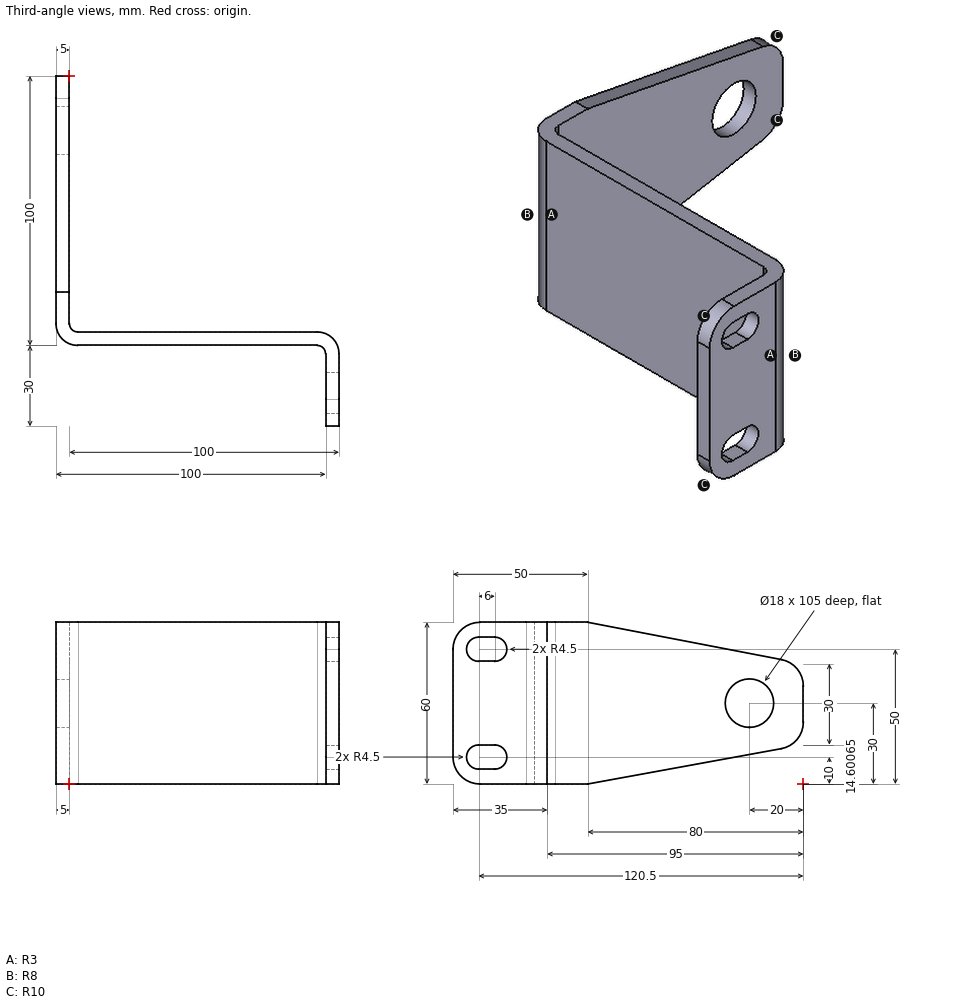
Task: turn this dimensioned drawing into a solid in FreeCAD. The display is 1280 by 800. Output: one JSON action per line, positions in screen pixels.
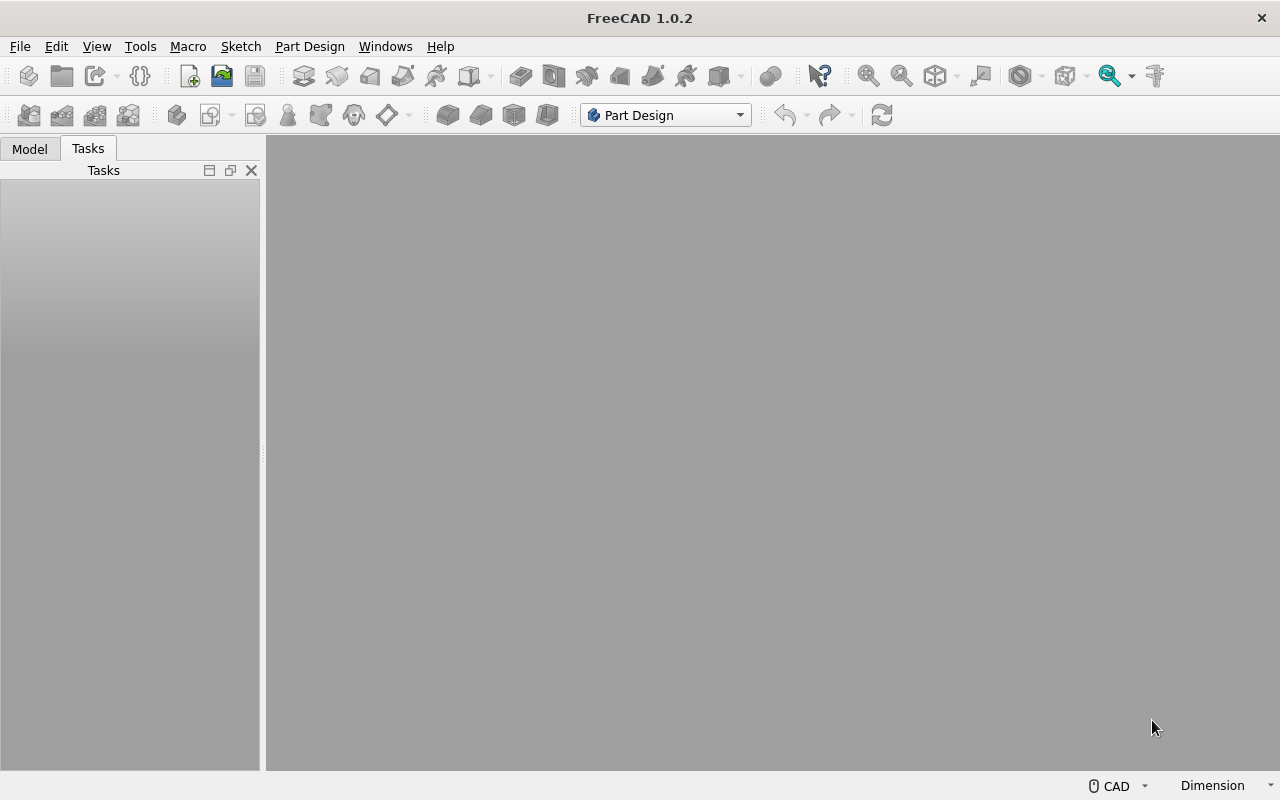
{"action": "left_click", "coordinate": [189, 76]}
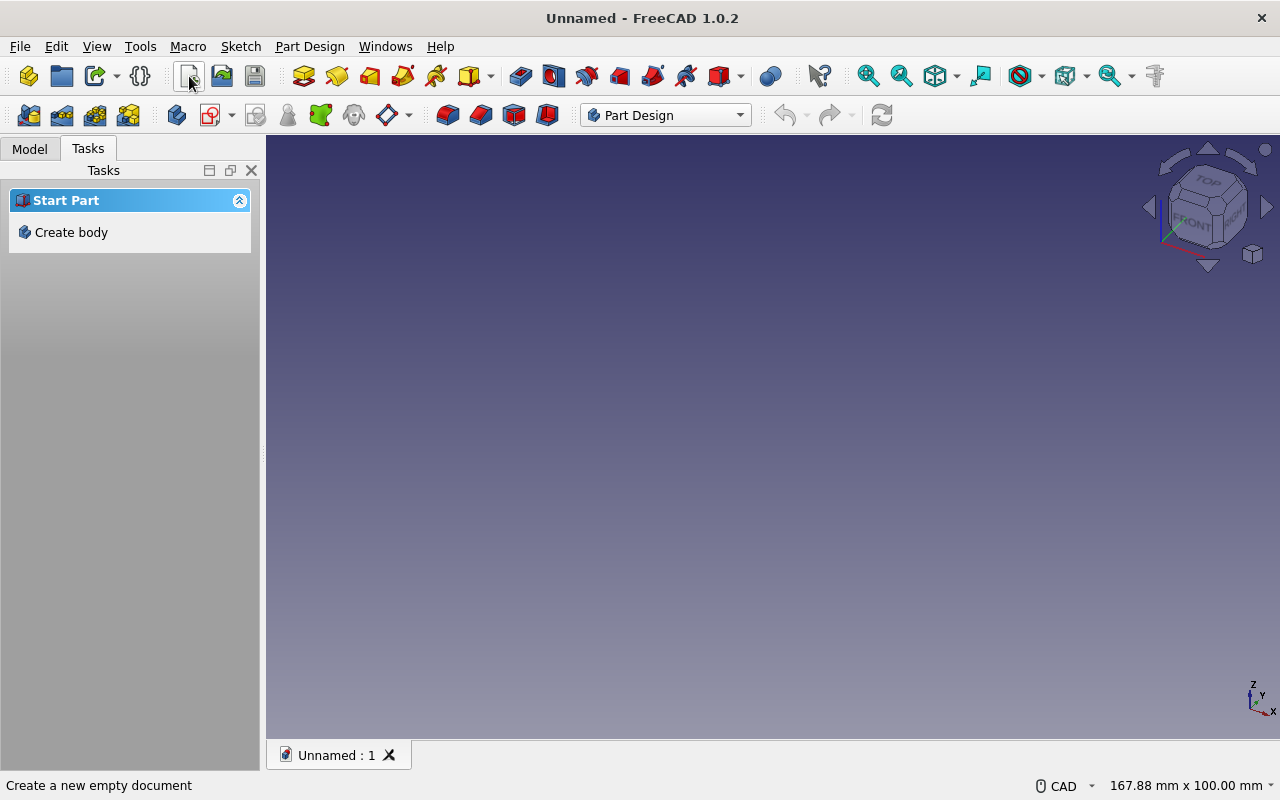
{"action": "left_click", "coordinate": [210, 116]}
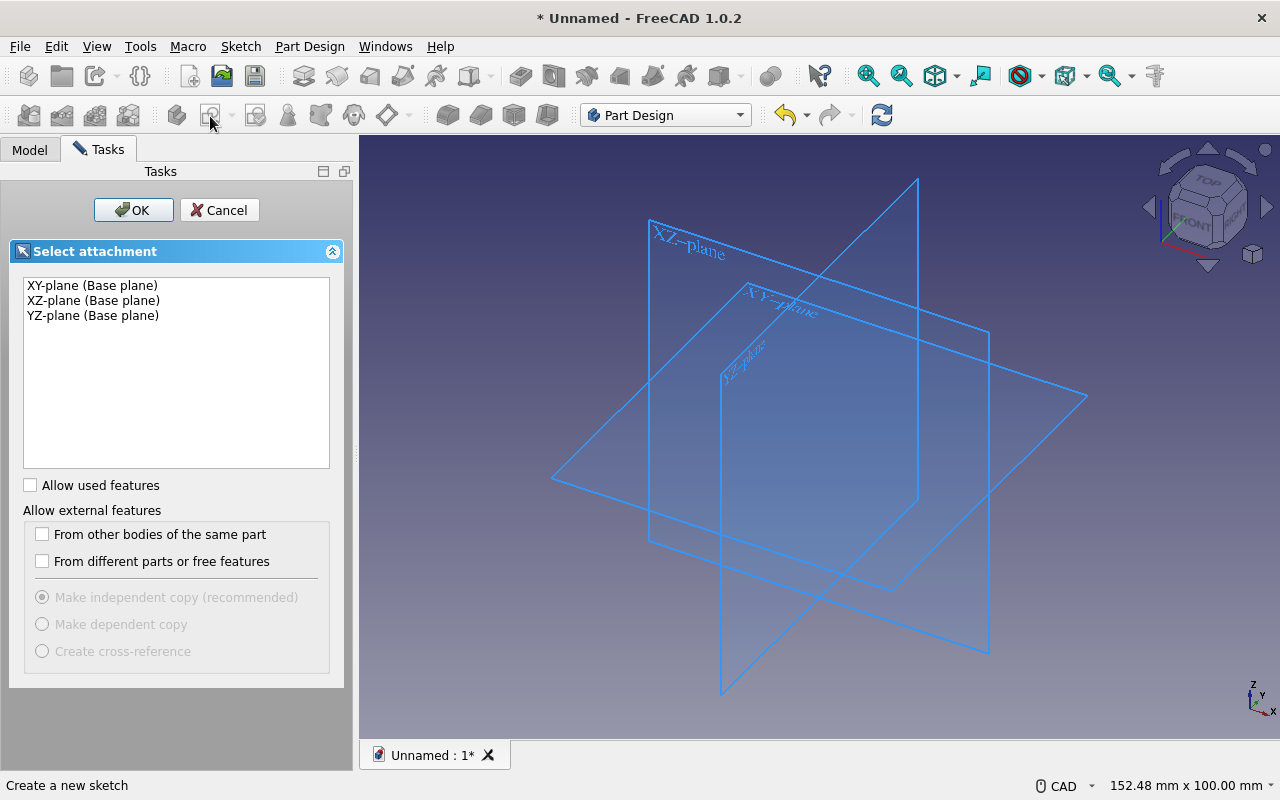
{"action": "left_click", "coordinate": [84, 316]}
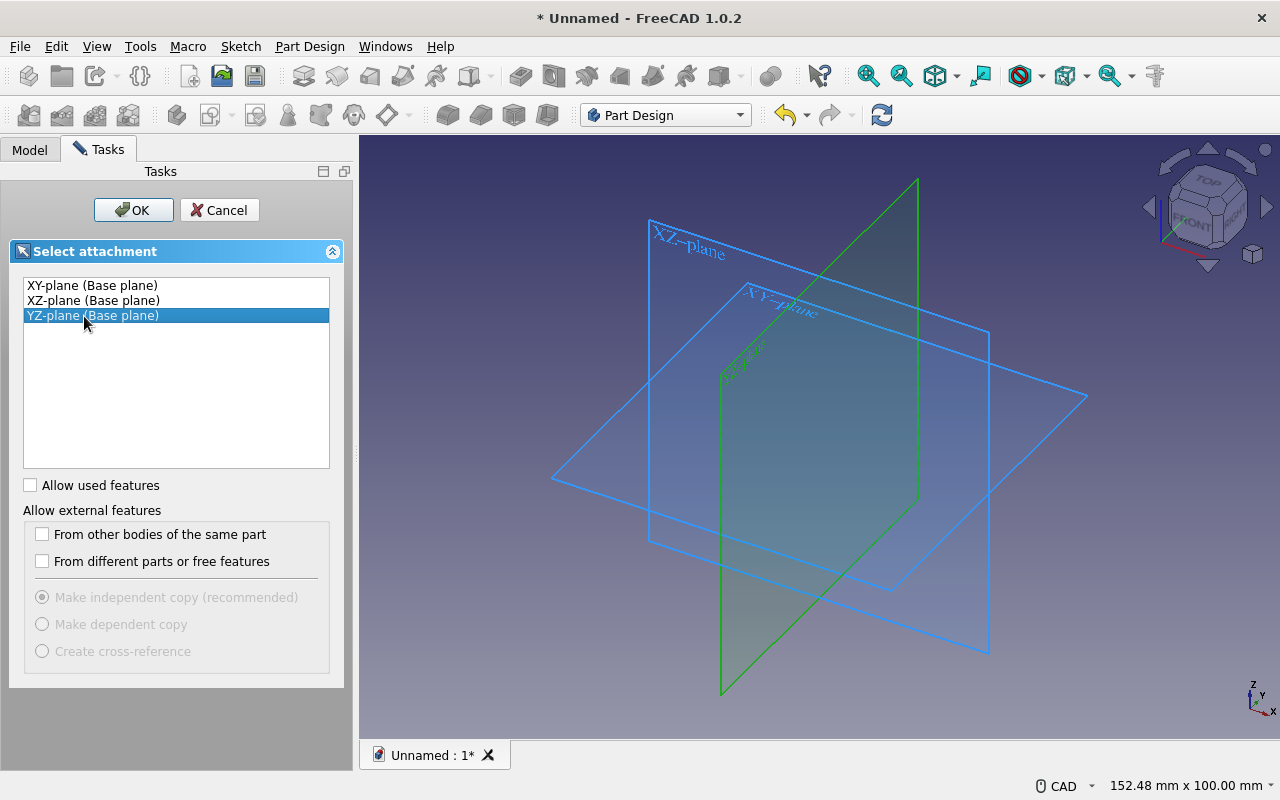
{"action": "left_click", "coordinate": [134, 210]}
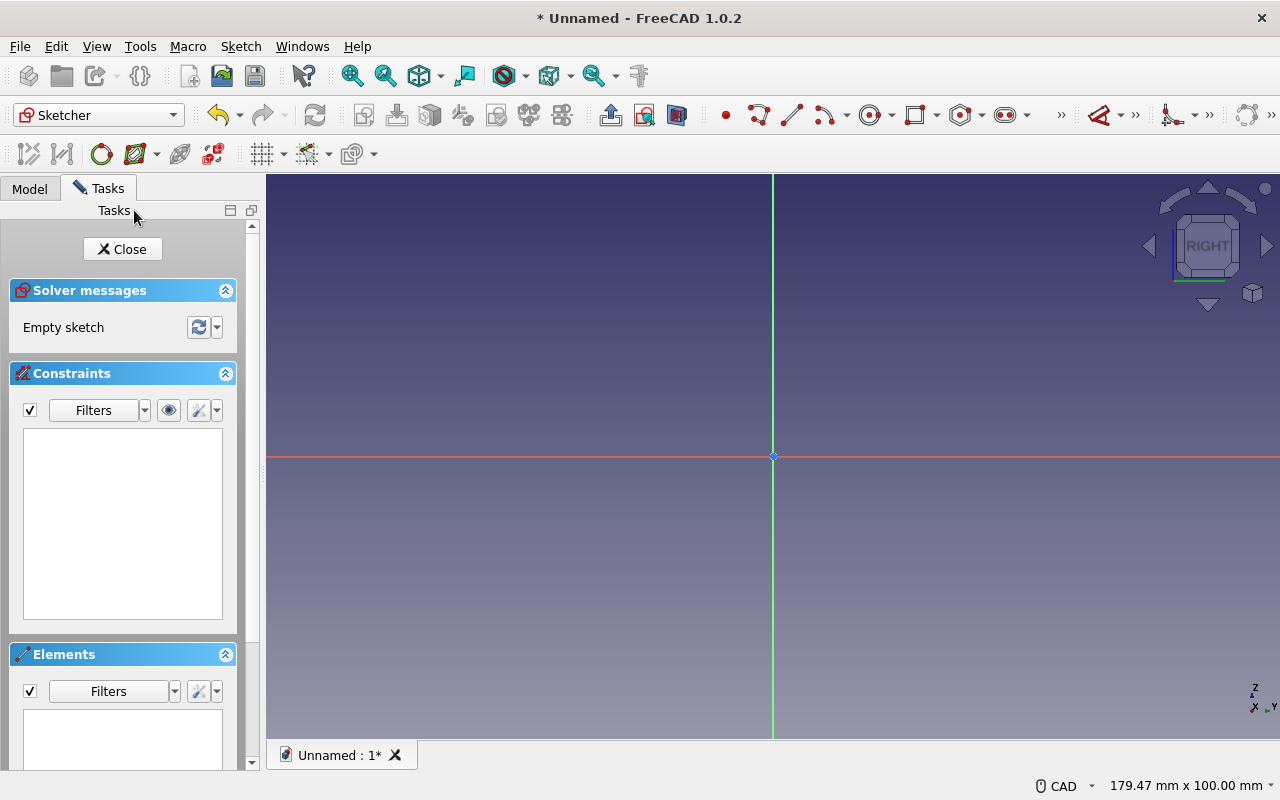
{"action": "scroll", "coordinate": [1115, 711], "scroll_direction": "down", "scroll_amount": 2}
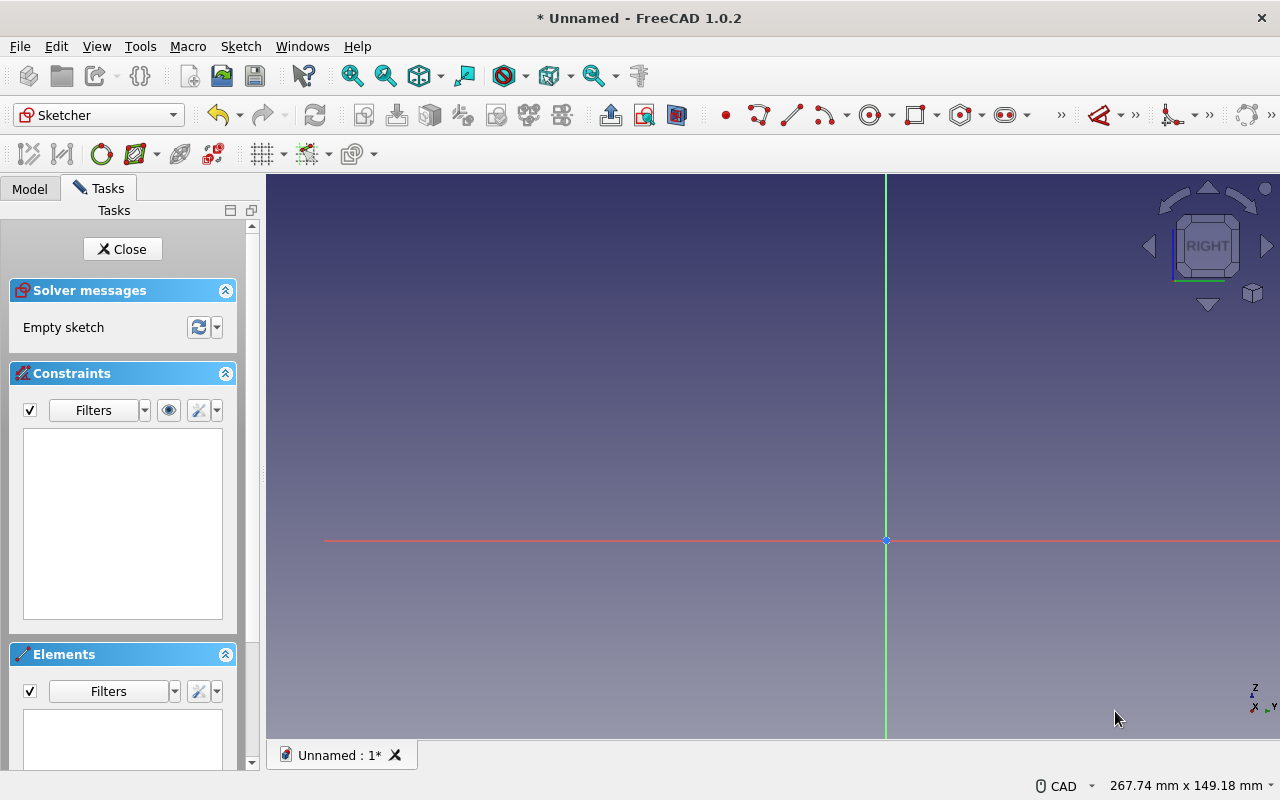
{"action": "left_click", "coordinate": [759, 116]}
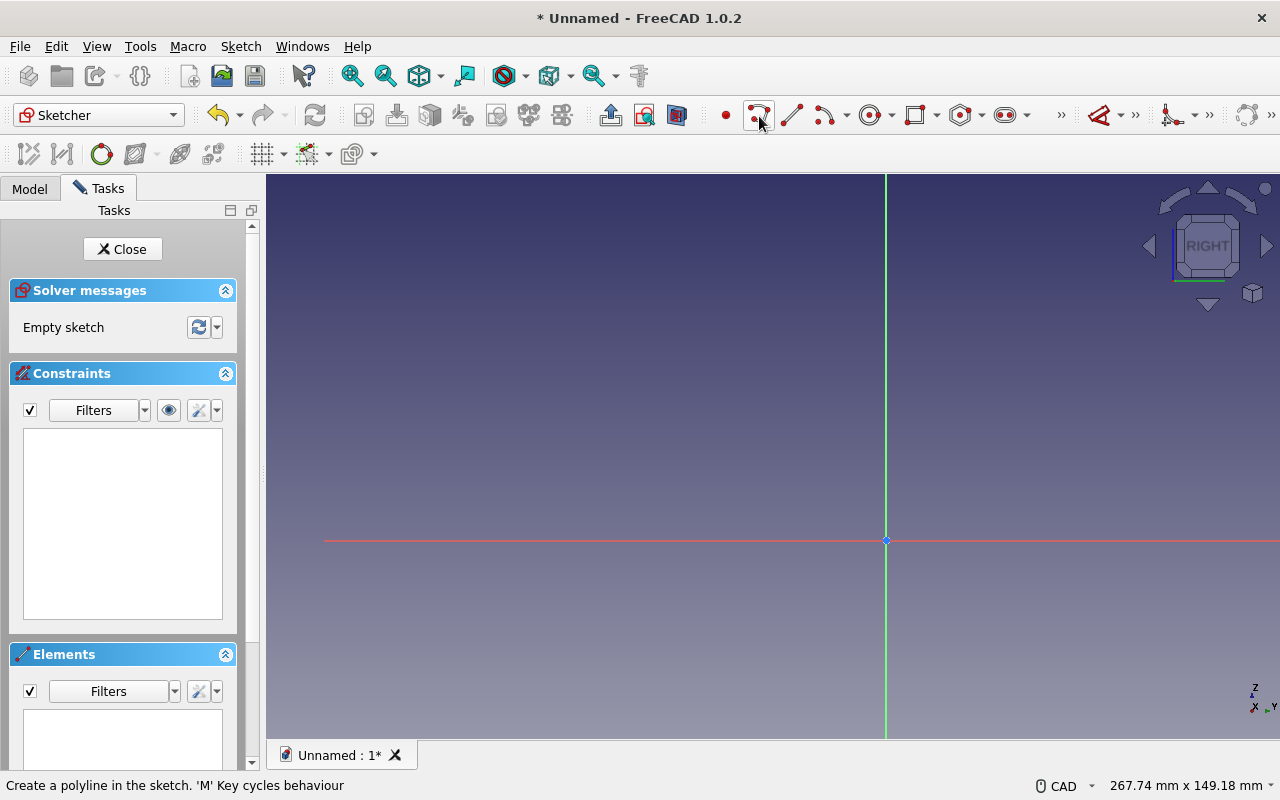
{"action": "left_click", "coordinate": [886, 485]}
{"action": "left_click", "coordinate": [877, 372]}
{"action": "left_click", "coordinate": [583, 313]}
{"action": "left_click", "coordinate": [394, 313]}
{"action": "left_click", "coordinate": [394, 541]}
{"action": "left_click", "coordinate": [583, 532]}
{"action": "left_click", "coordinate": [886, 486]}
{"action": "key", "text": "Escape"}
{"action": "key", "text": "Escape"}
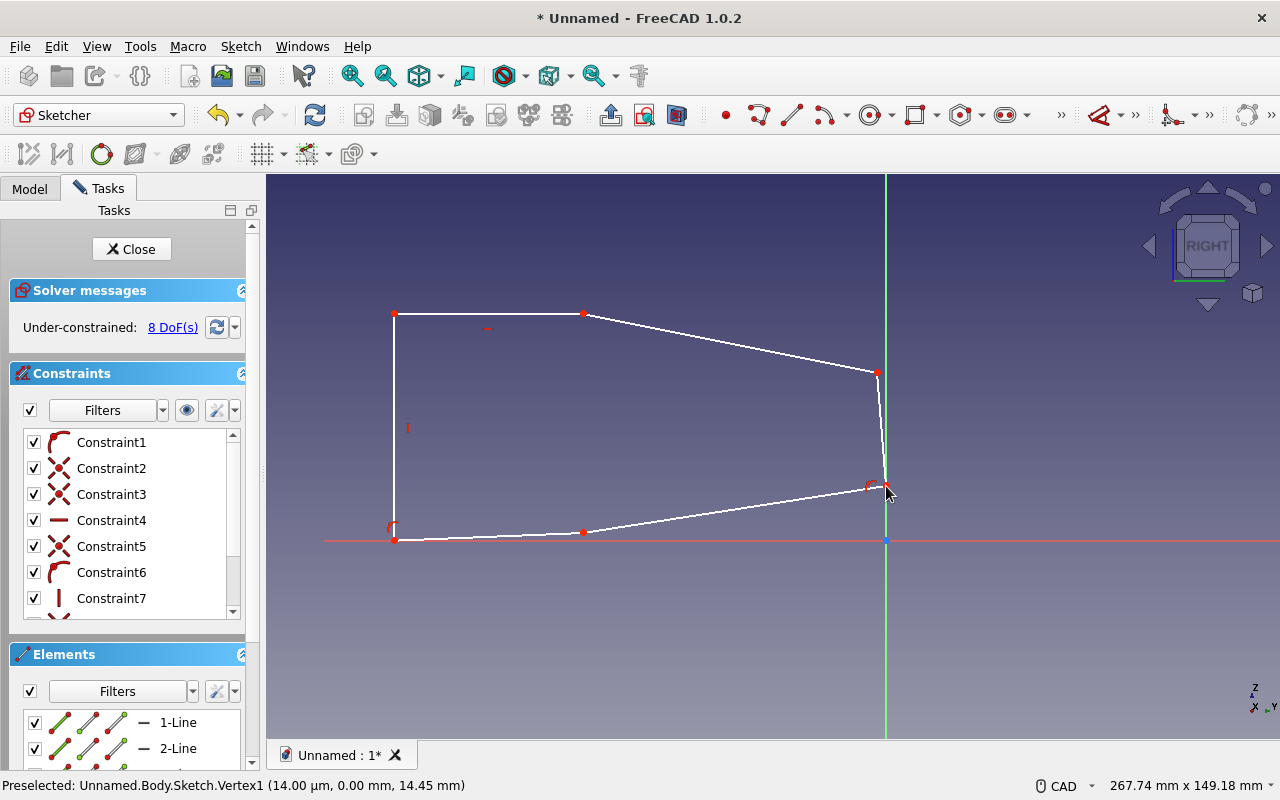
{"action": "left_click", "coordinate": [883, 452]}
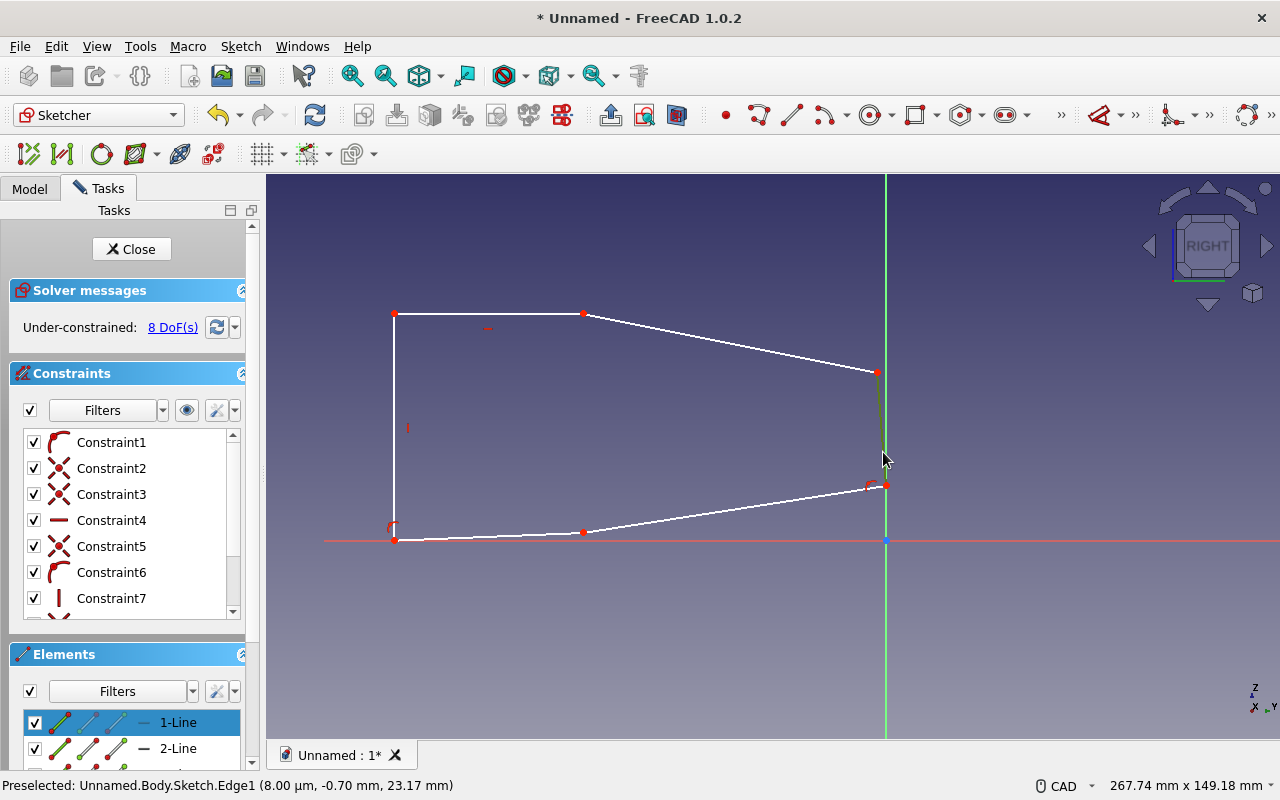
{"action": "key", "text": "v"}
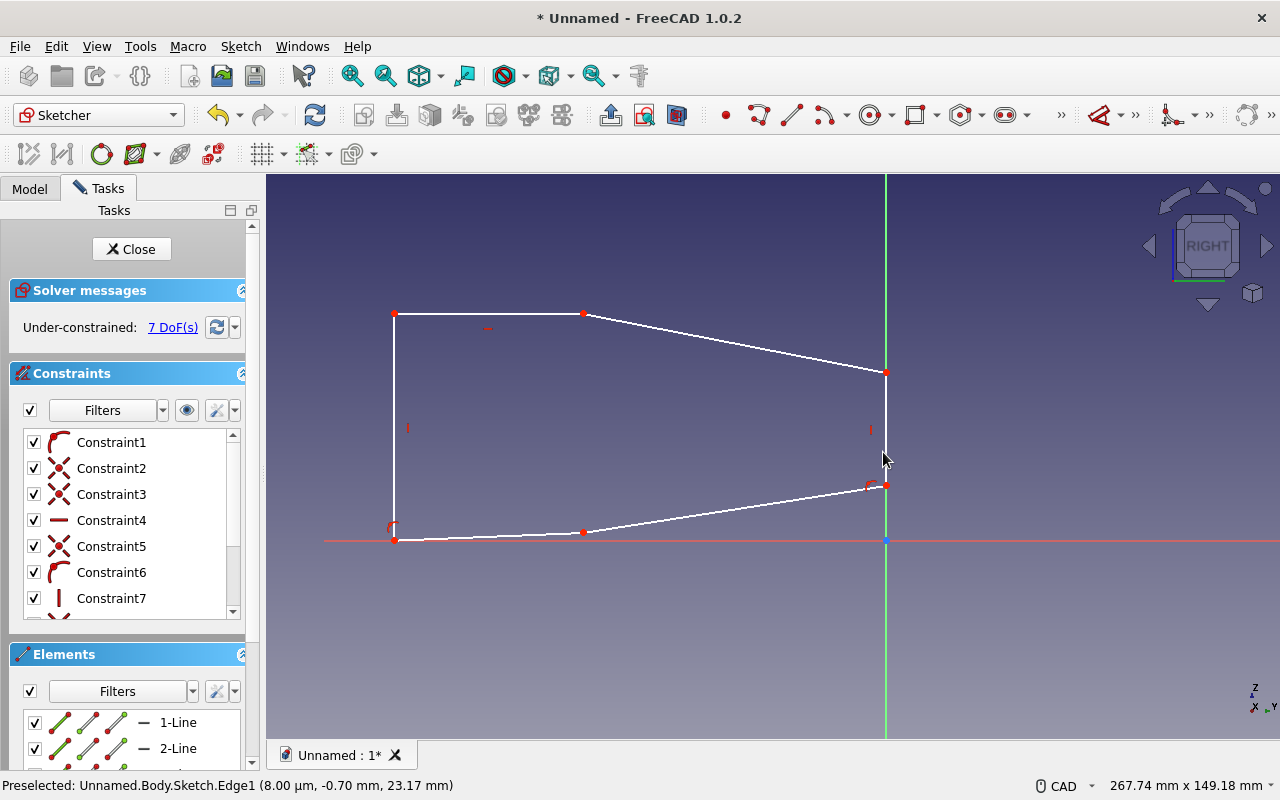
{"action": "left_click", "coordinate": [451, 538]}